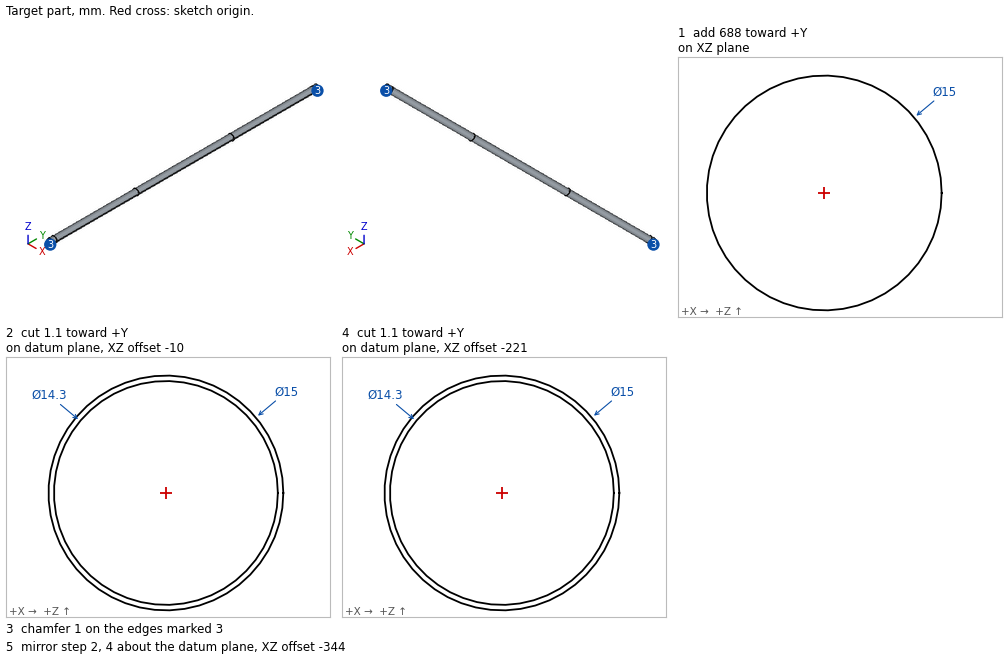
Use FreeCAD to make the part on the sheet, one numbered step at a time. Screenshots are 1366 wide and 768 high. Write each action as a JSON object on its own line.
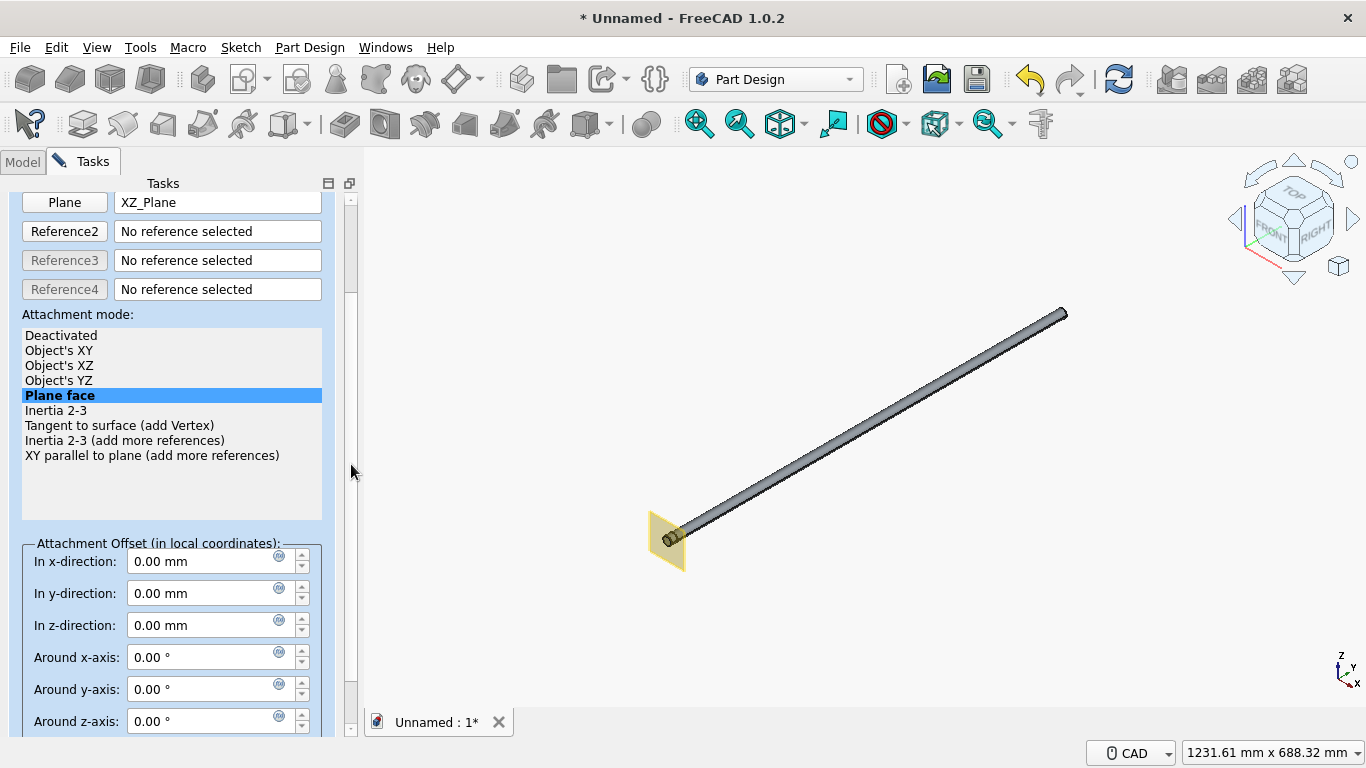
{"action": "triple_click", "coordinate": [210, 625]}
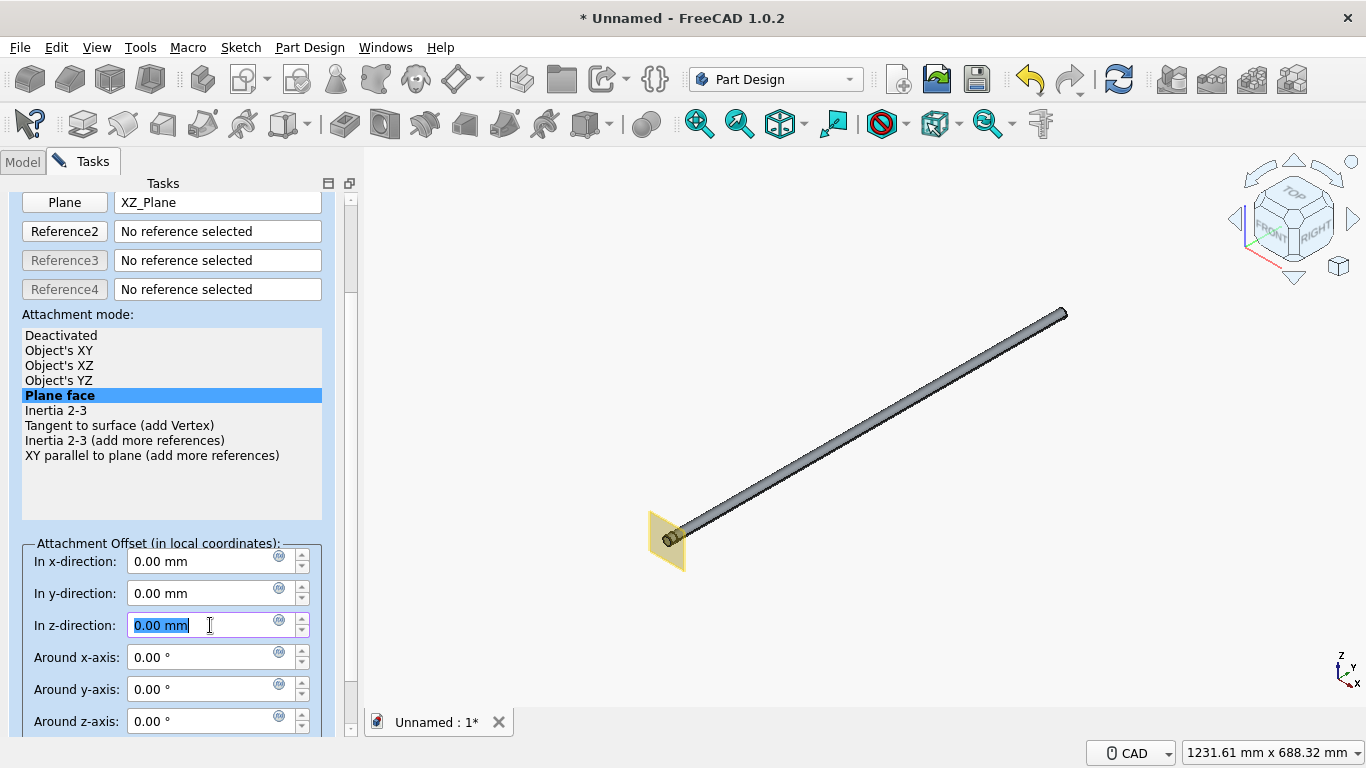
{"action": "type", "text": "-221"}
{"action": "key", "text": "Tab"}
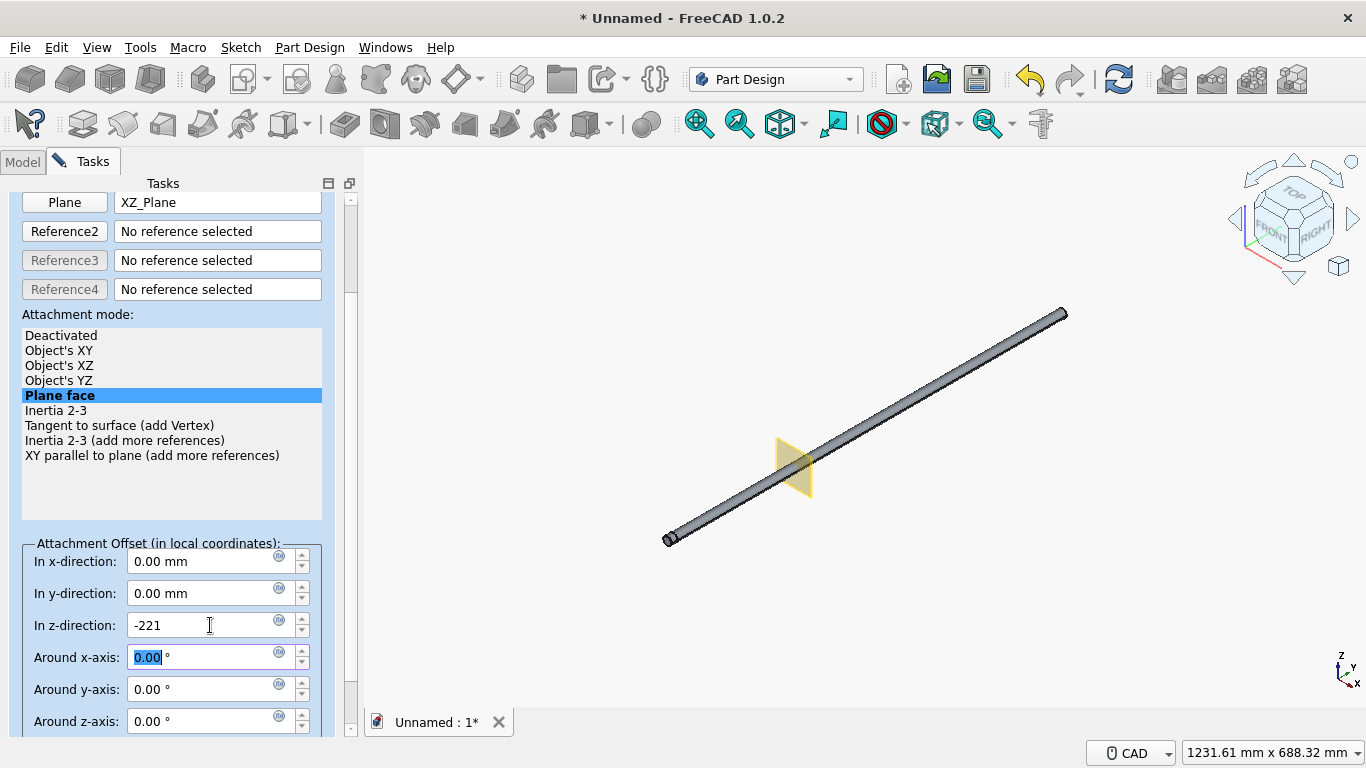
{"action": "scroll", "coordinate": [351, 464], "scroll_direction": "up", "scroll_amount": 3}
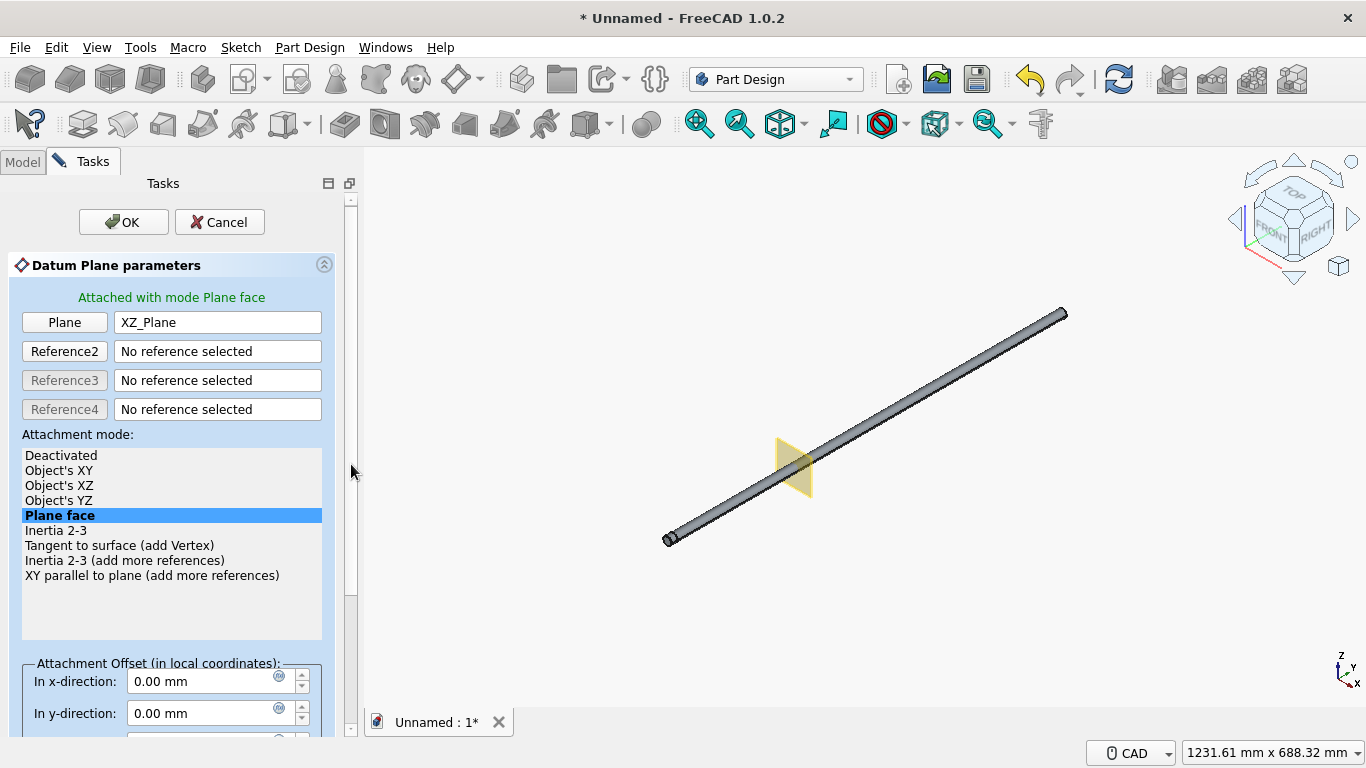
{"action": "left_click", "coordinate": [124, 222]}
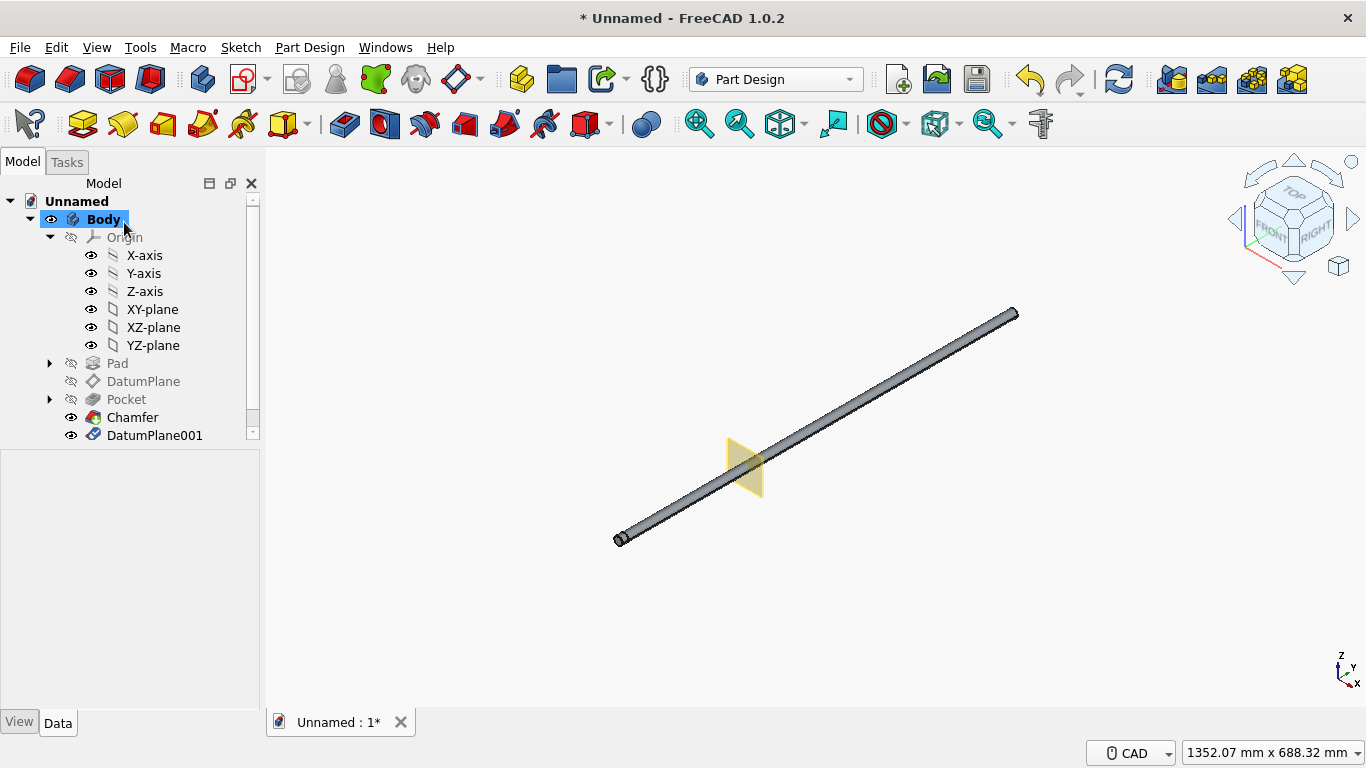
{"action": "left_click", "coordinate": [116, 435]}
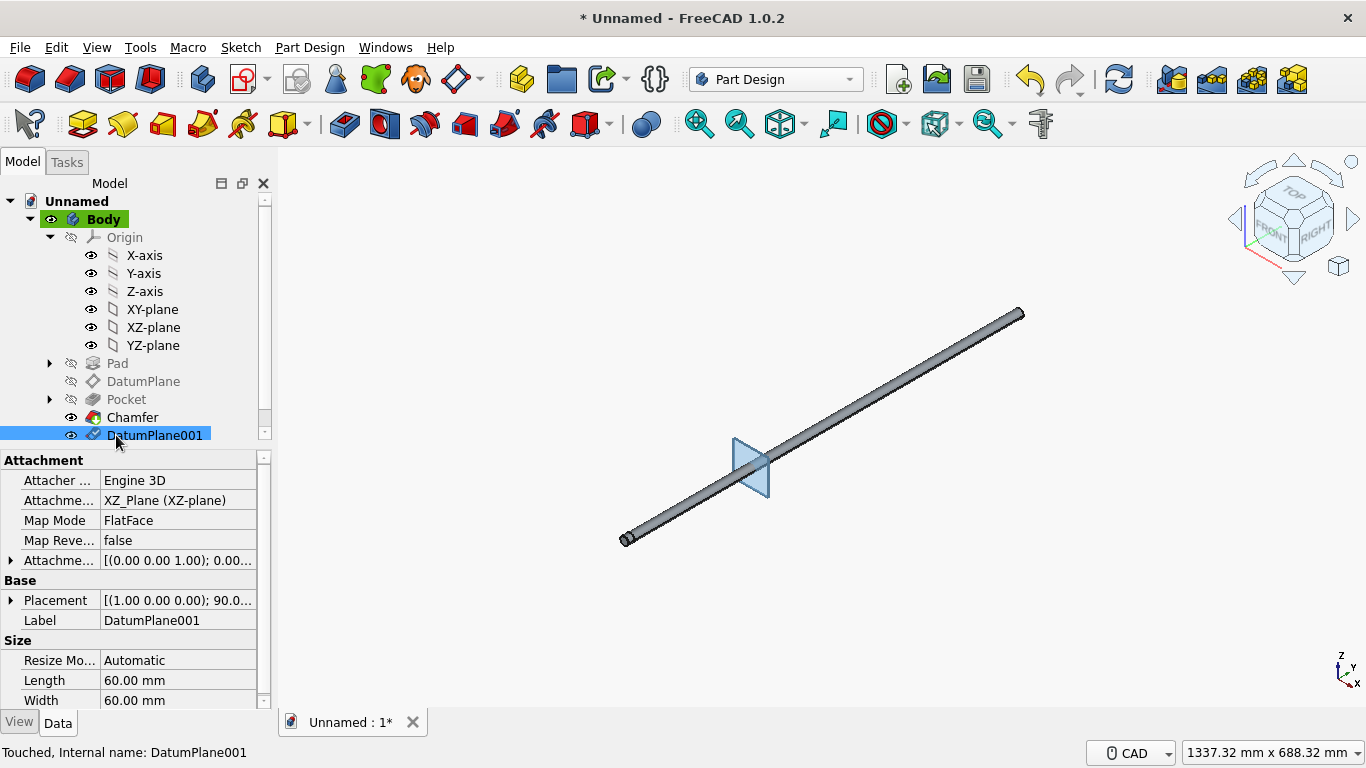
{"action": "left_click", "coordinate": [244, 80]}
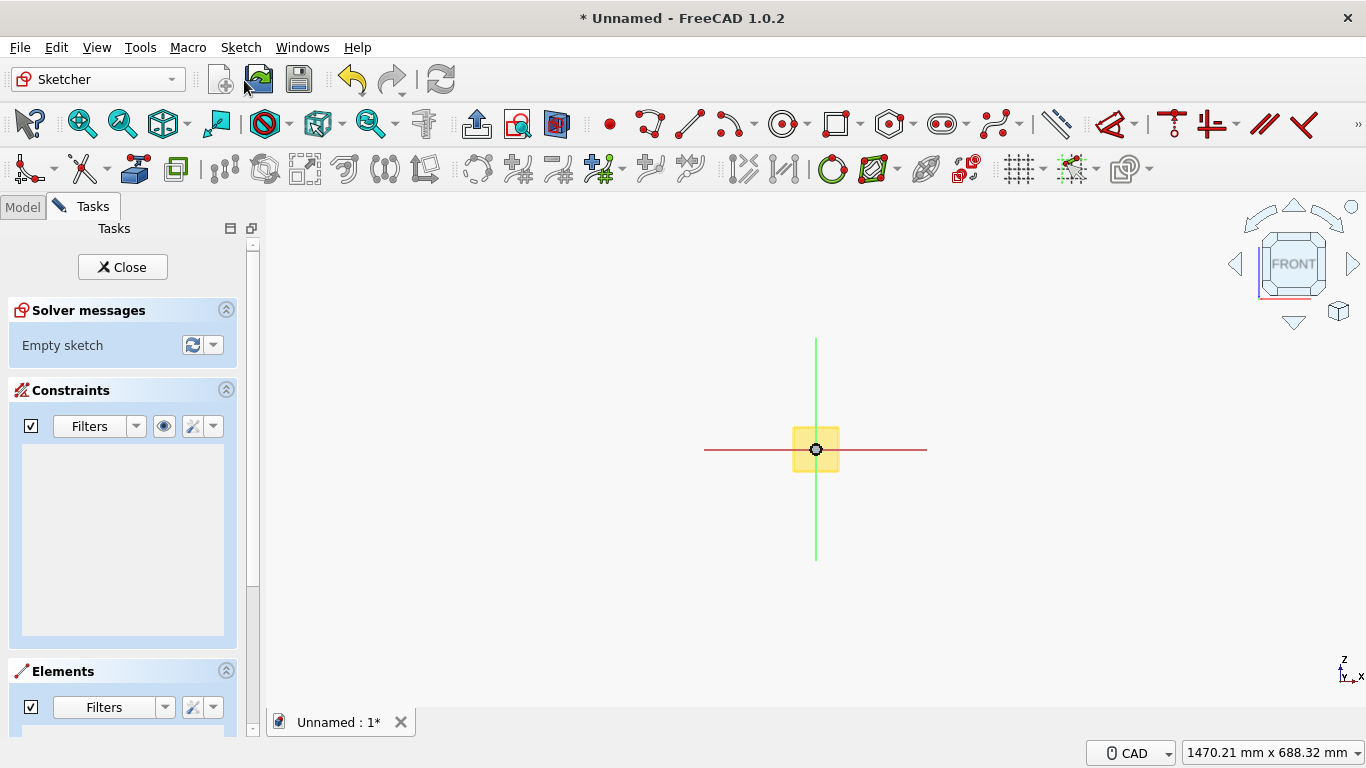
{"action": "left_click", "coordinate": [558, 124]}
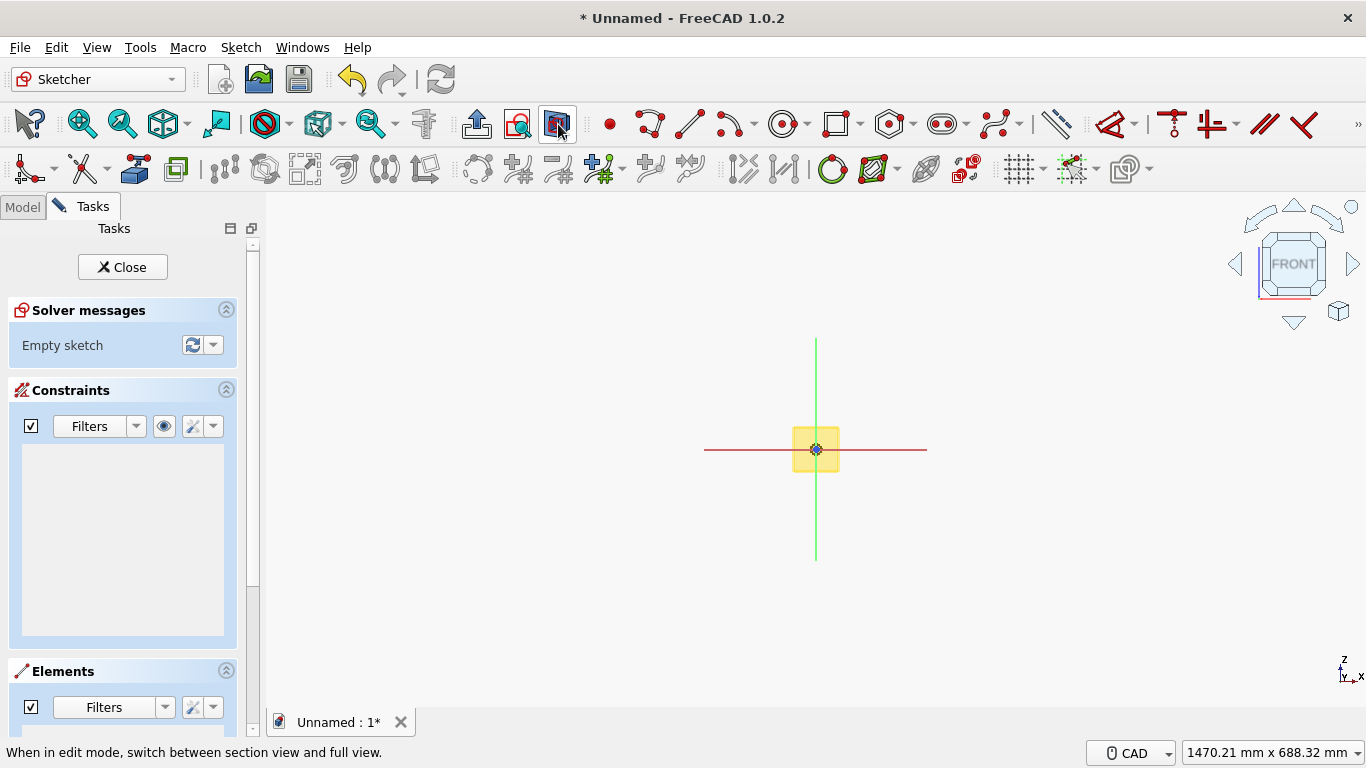
{"action": "scroll", "coordinate": [820, 450], "scroll_direction": "up", "scroll_amount": 15}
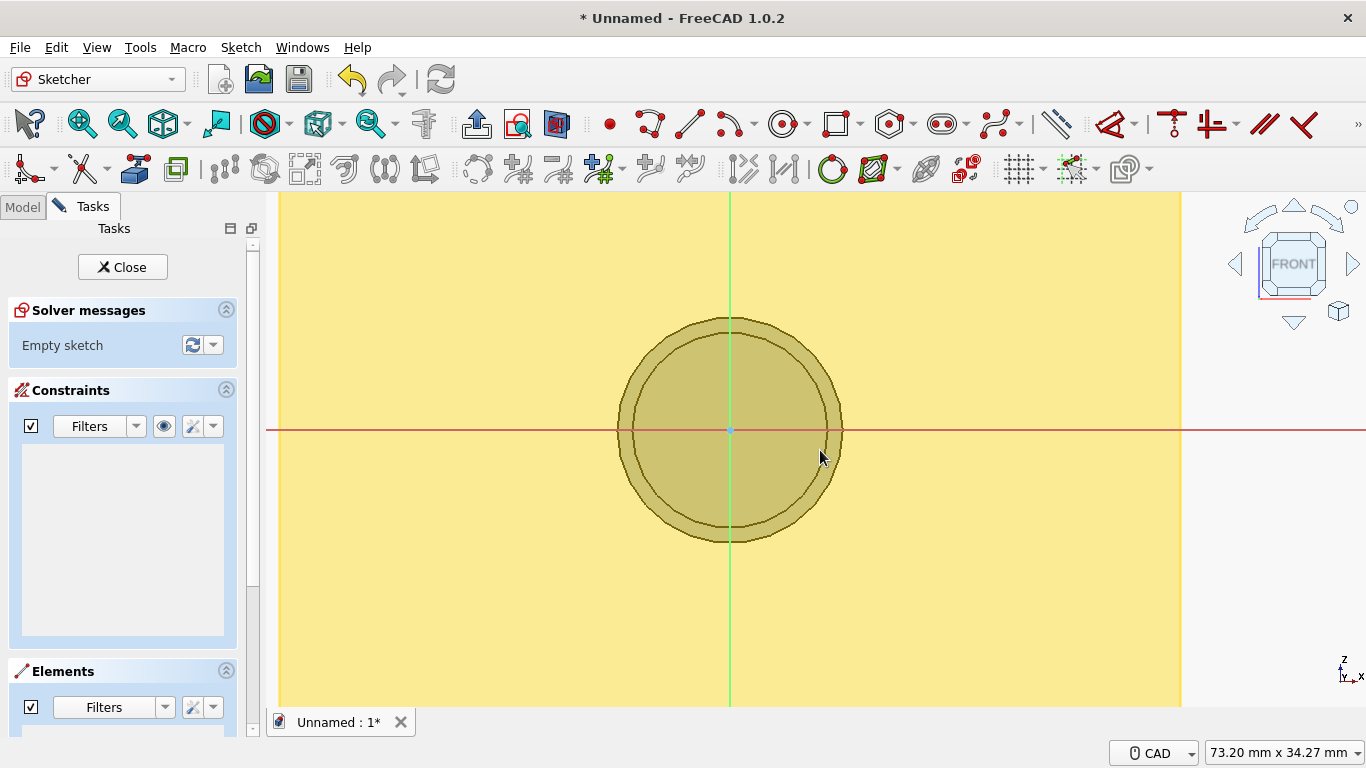
{"action": "scroll", "coordinate": [695, 391], "scroll_direction": "up", "scroll_amount": 2}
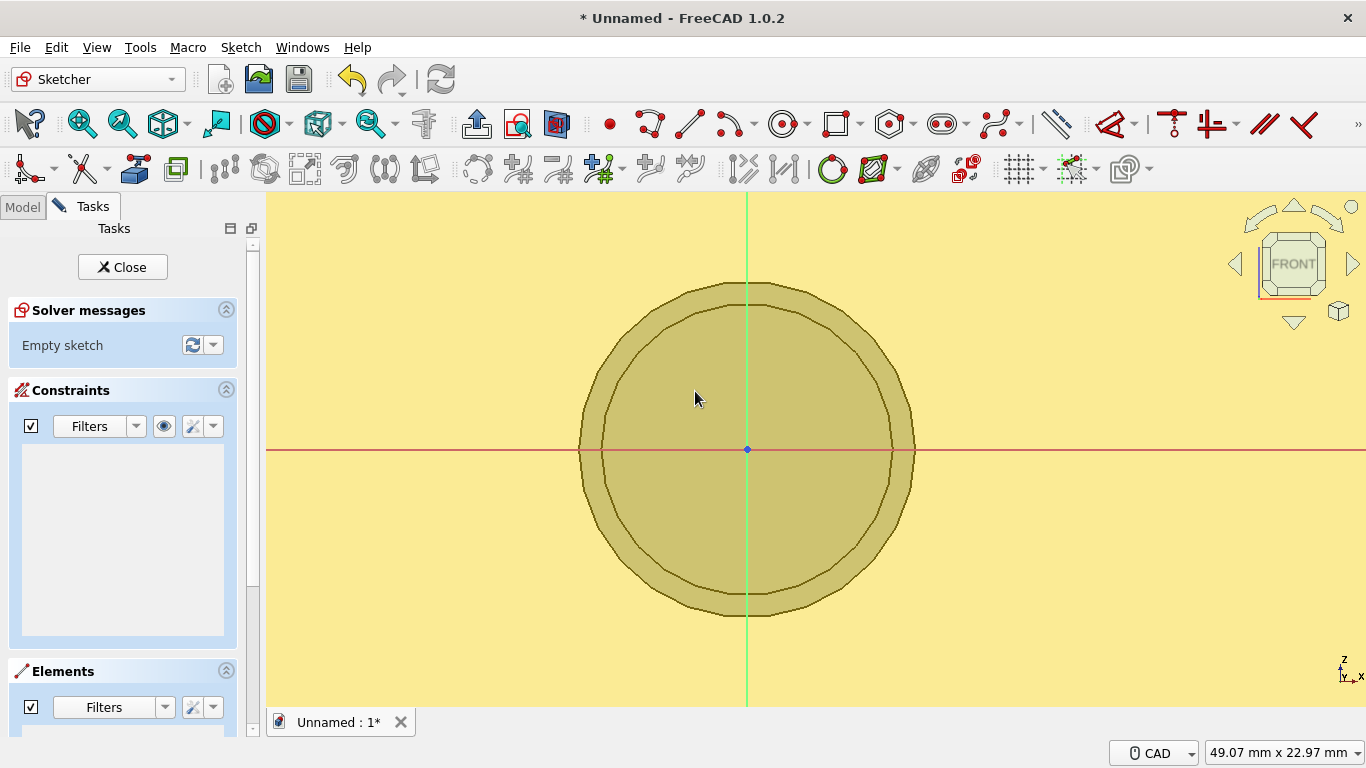
{"action": "left_click", "coordinate": [784, 124]}